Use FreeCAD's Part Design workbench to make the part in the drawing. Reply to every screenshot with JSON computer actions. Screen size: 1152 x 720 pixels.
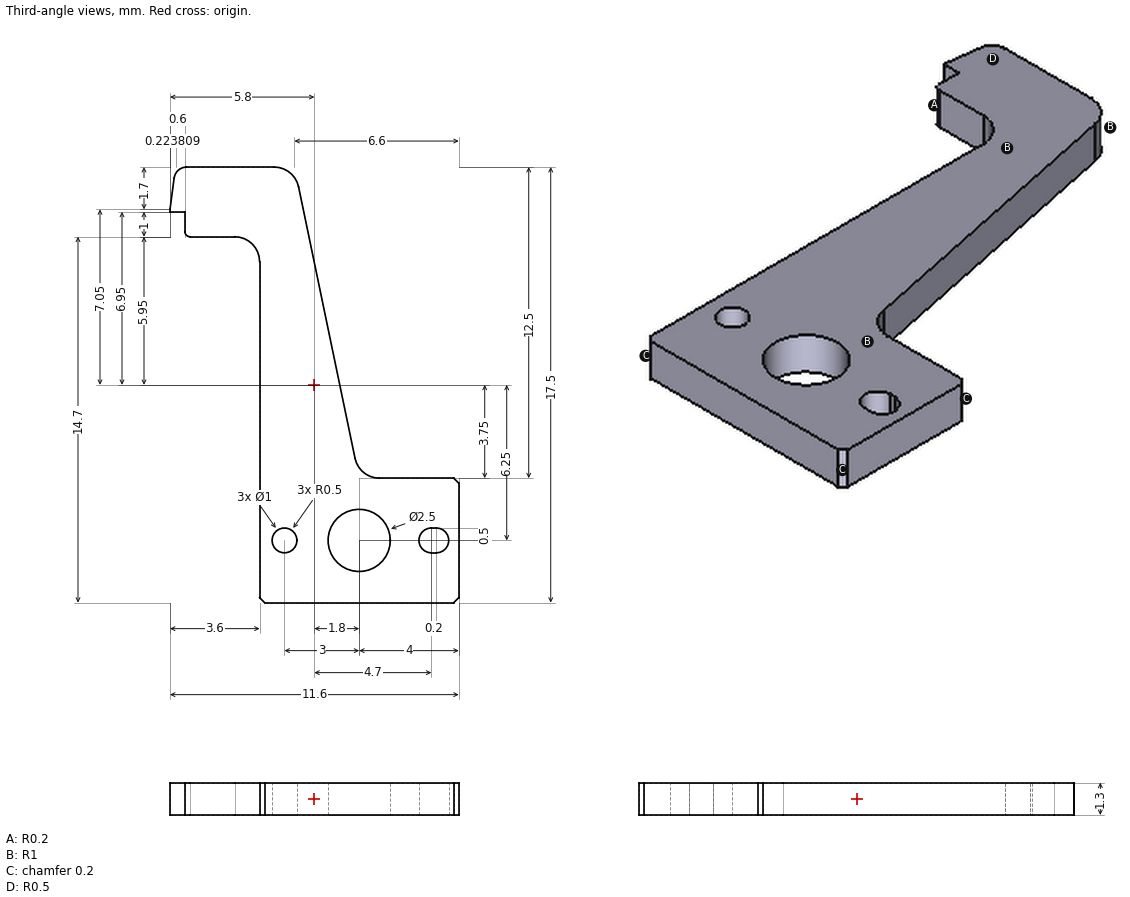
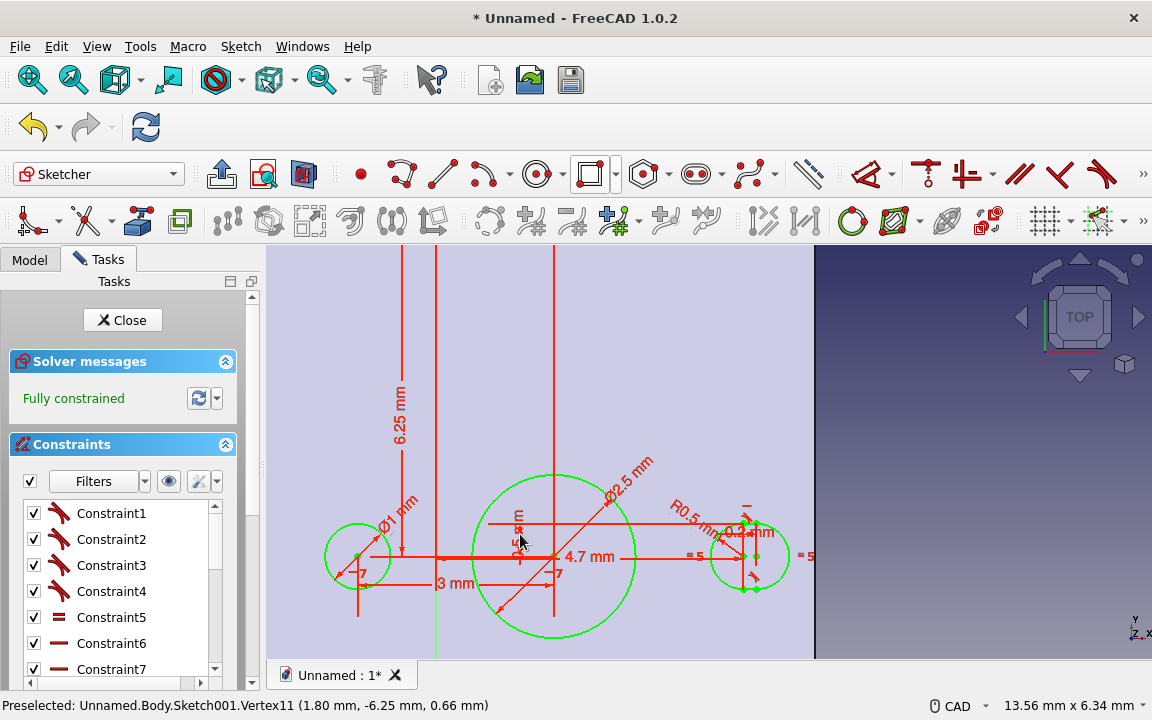
{"action": "left_click", "coordinate": [123, 320]}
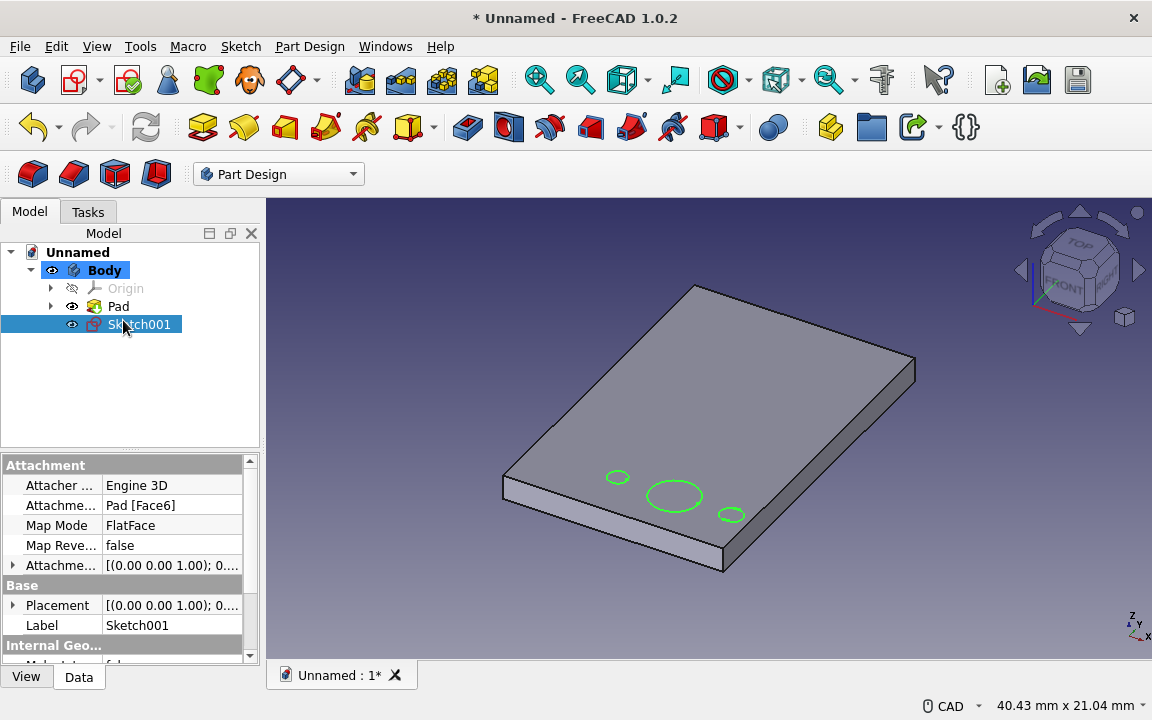
{"action": "left_click", "coordinate": [468, 128]}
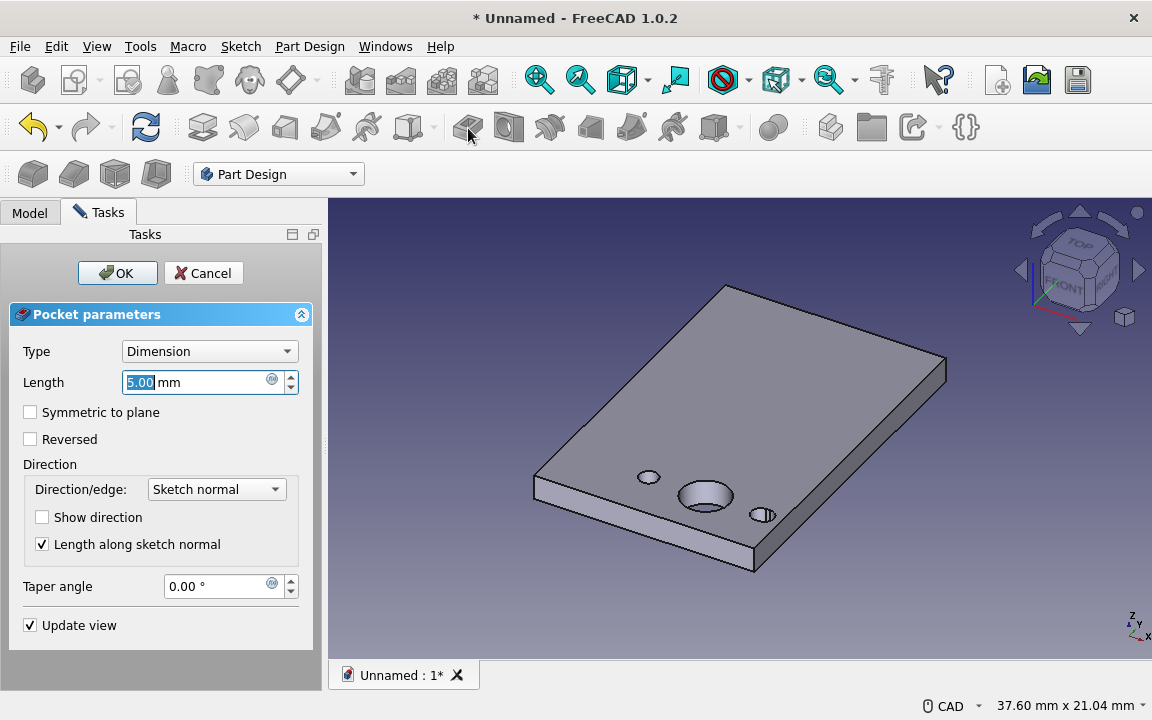
{"action": "left_click", "coordinate": [210, 352]}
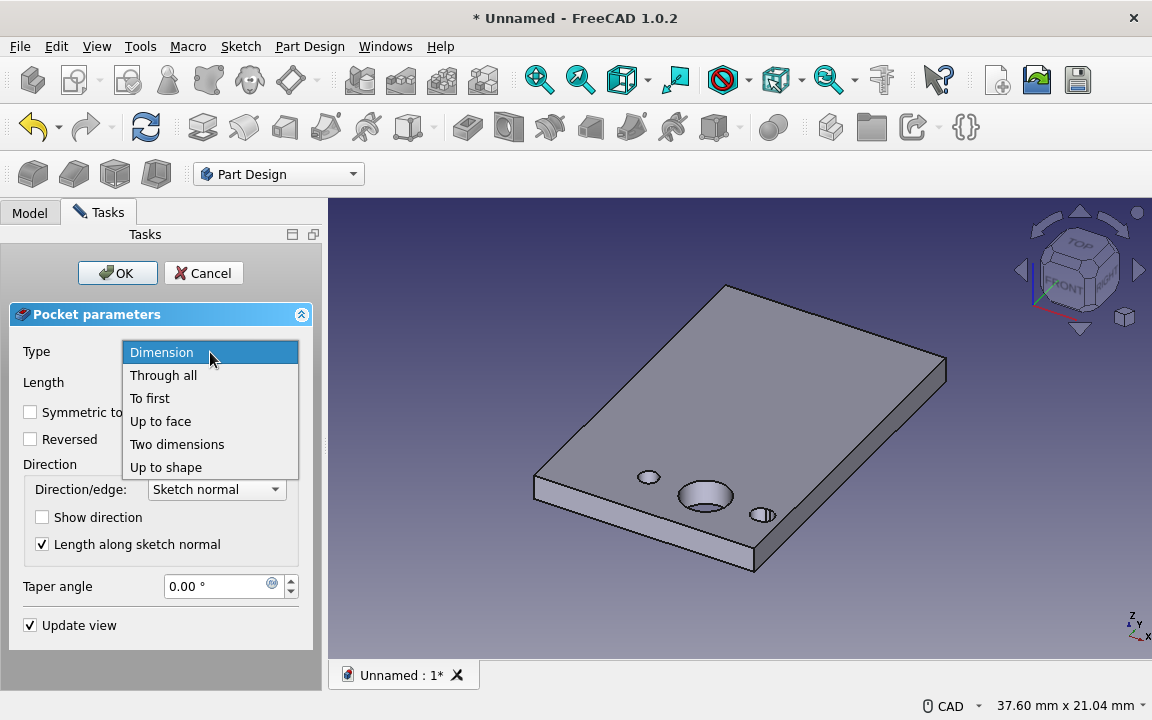
{"action": "left_click", "coordinate": [208, 376]}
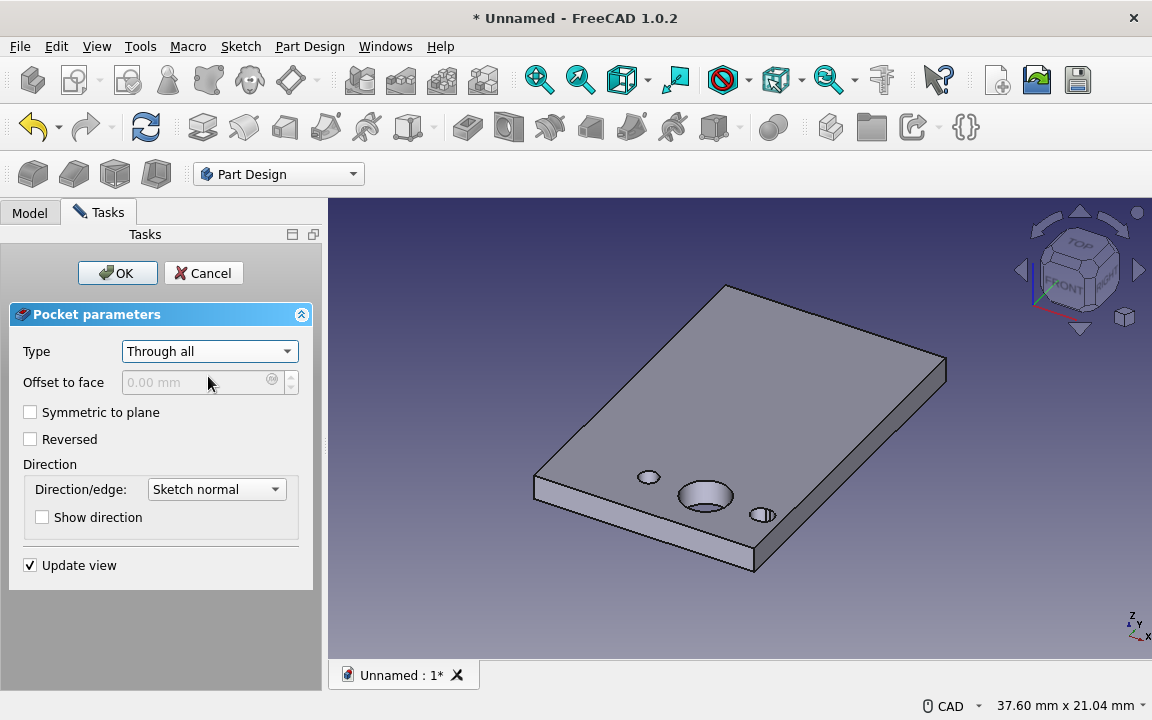
{"action": "left_click", "coordinate": [118, 273]}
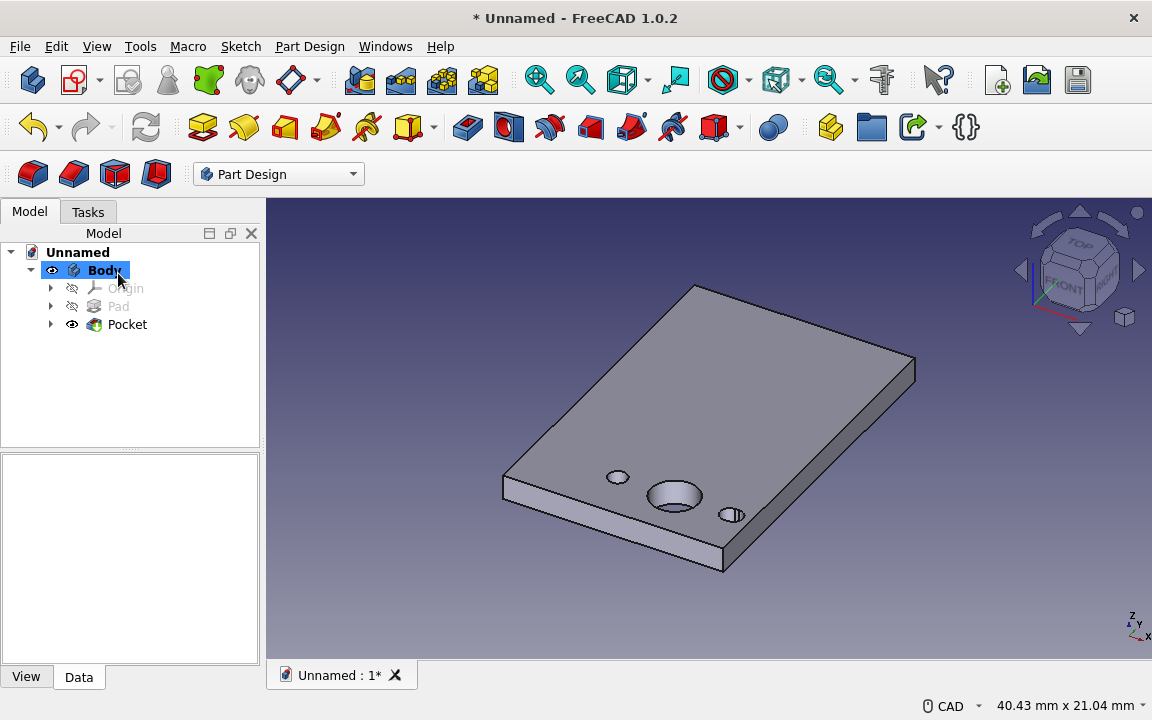
{"action": "left_click", "coordinate": [736, 389]}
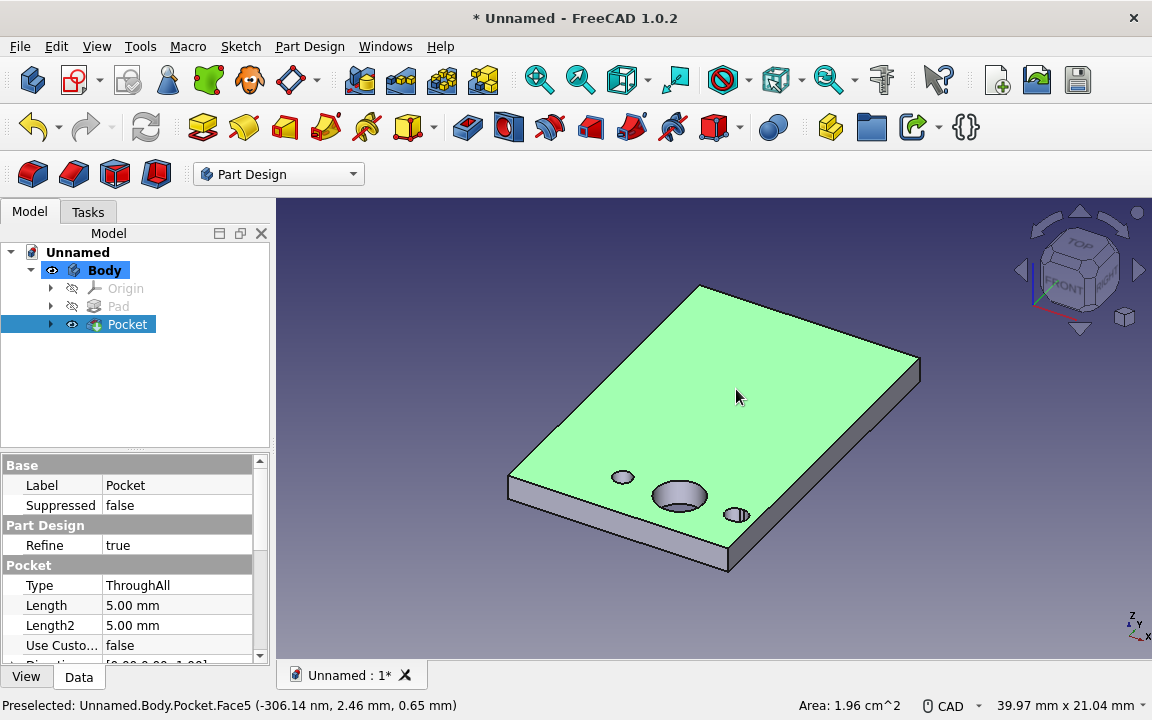
{"action": "left_click", "coordinate": [74, 80]}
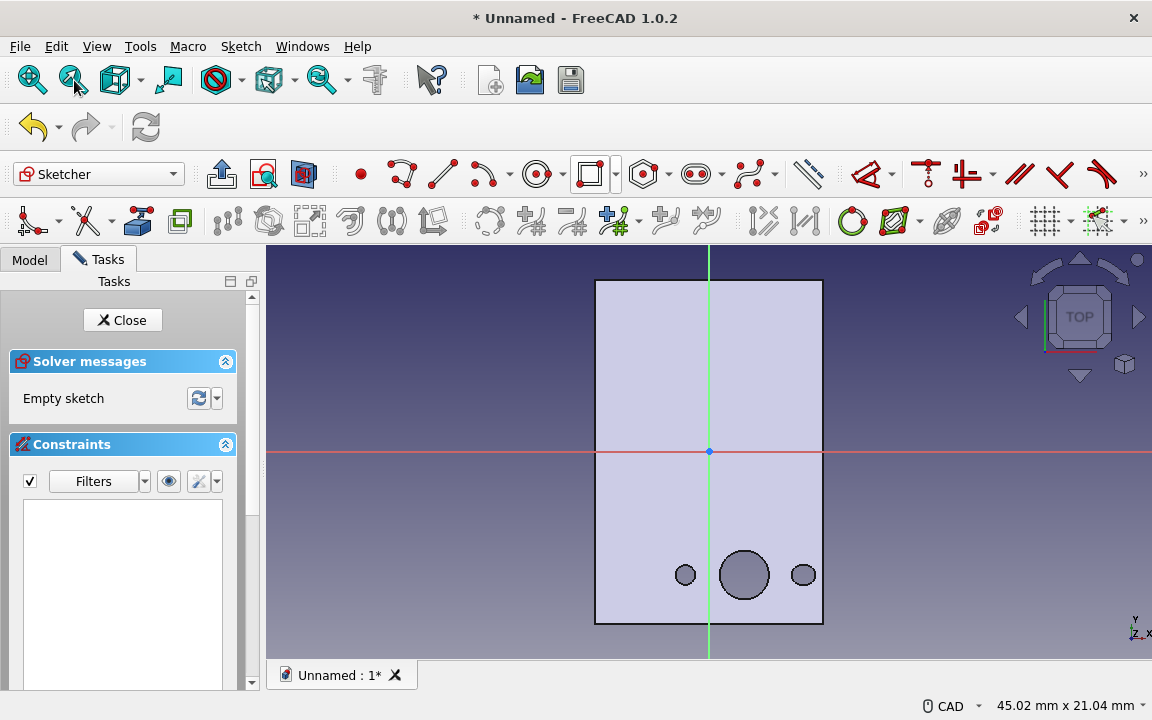
{"action": "scroll", "coordinate": [501, 452], "scroll_direction": "down", "scroll_amount": 2}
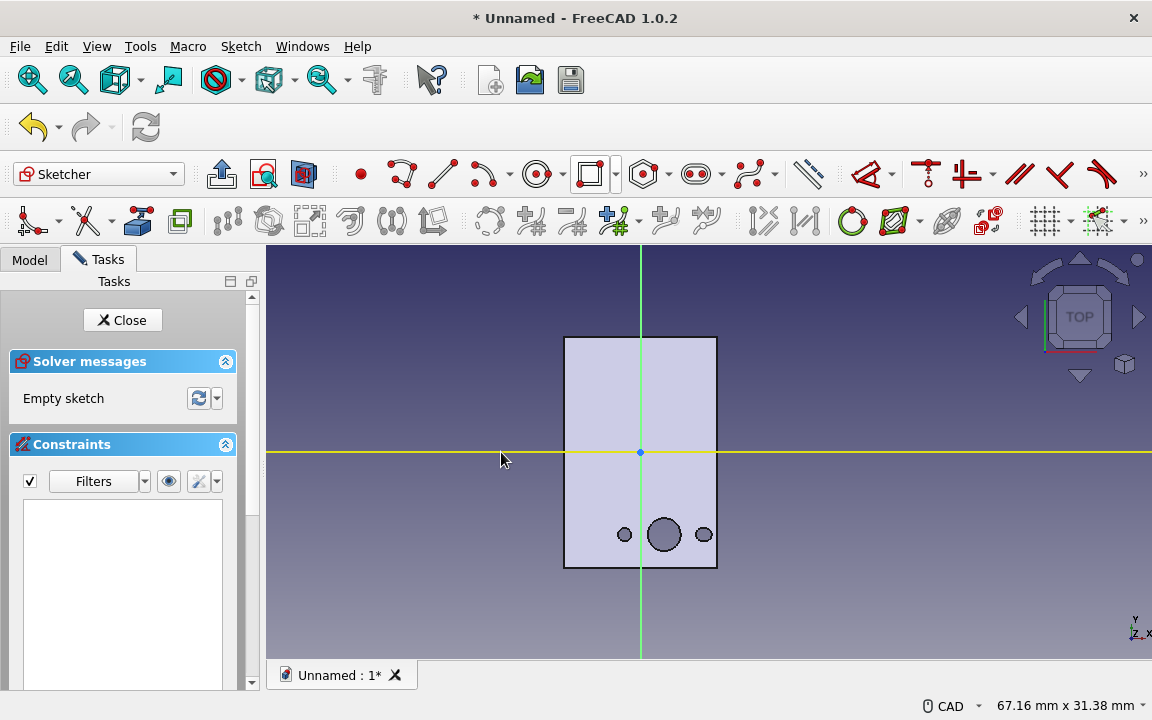
{"action": "key", "text": "g r"}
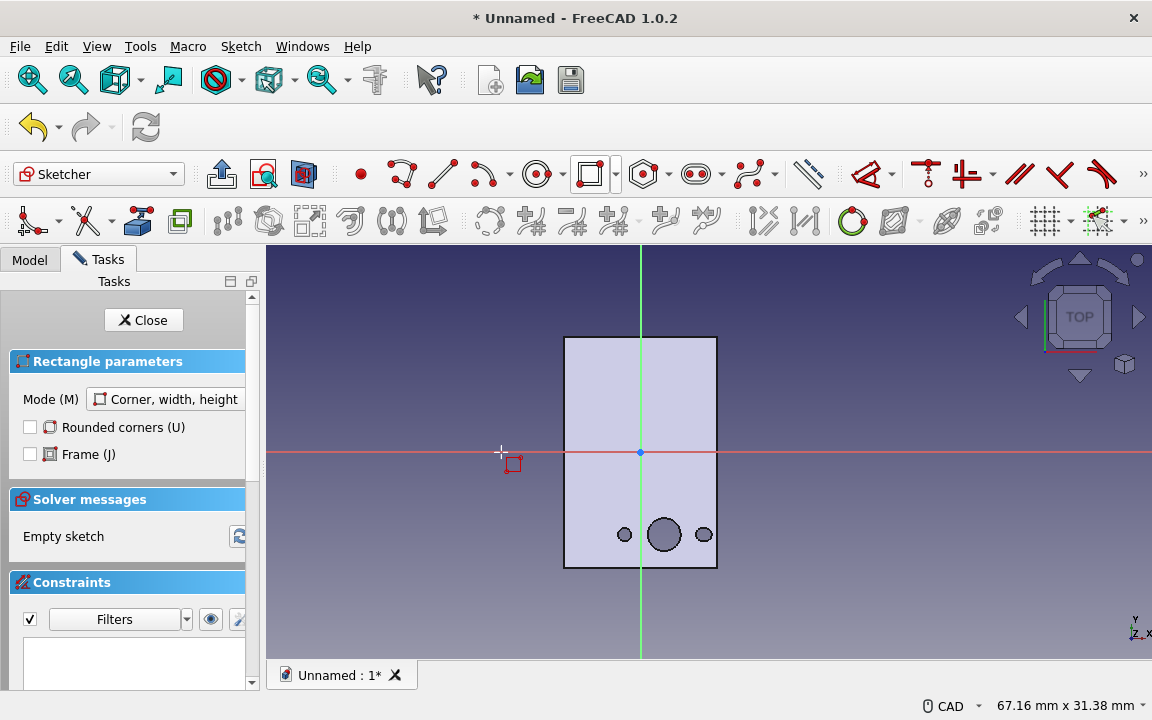
{"action": "left_click", "coordinate": [564, 374]}
{"action": "left_click", "coordinate": [611, 568]}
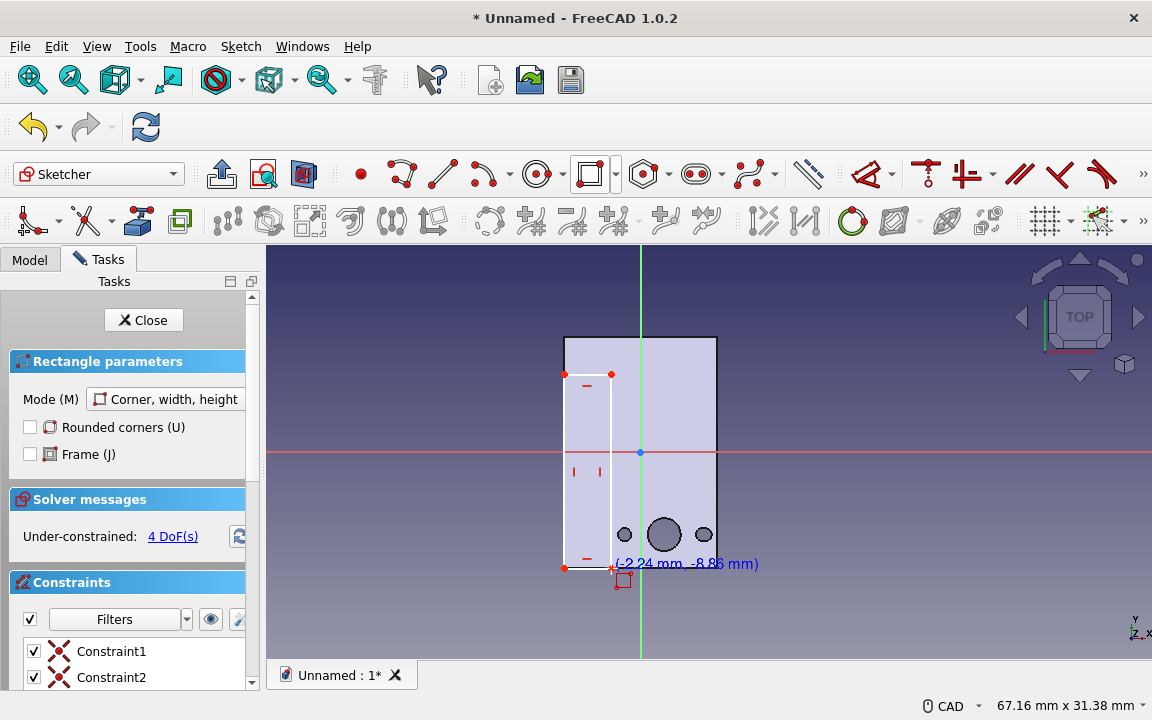
{"action": "left_click", "coordinate": [402, 174]}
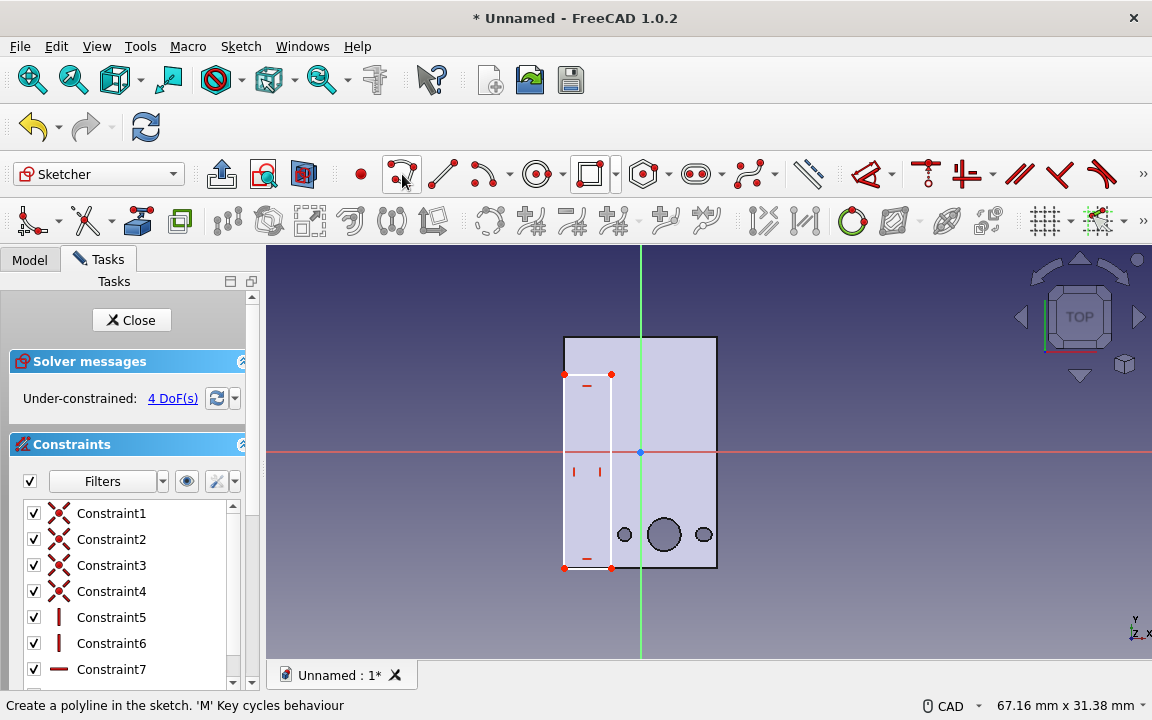
{"action": "left_click", "coordinate": [664, 502]}
{"action": "left_click", "coordinate": [717, 502]}
{"action": "left_click", "coordinate": [717, 337]}